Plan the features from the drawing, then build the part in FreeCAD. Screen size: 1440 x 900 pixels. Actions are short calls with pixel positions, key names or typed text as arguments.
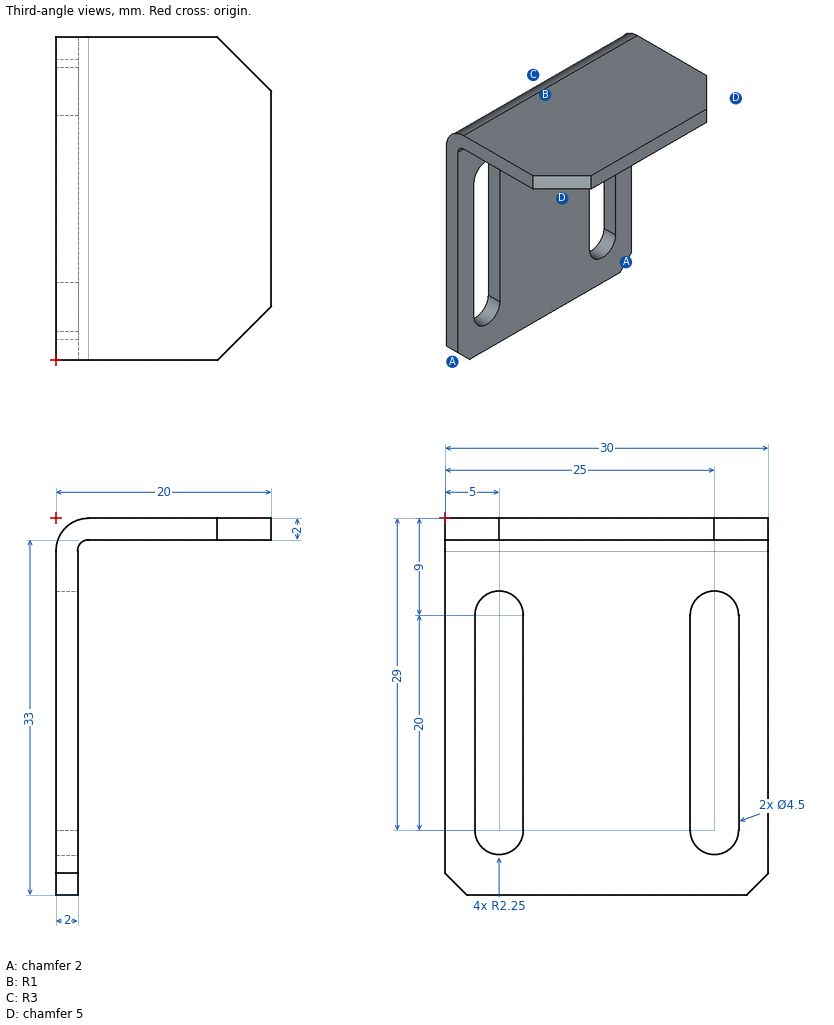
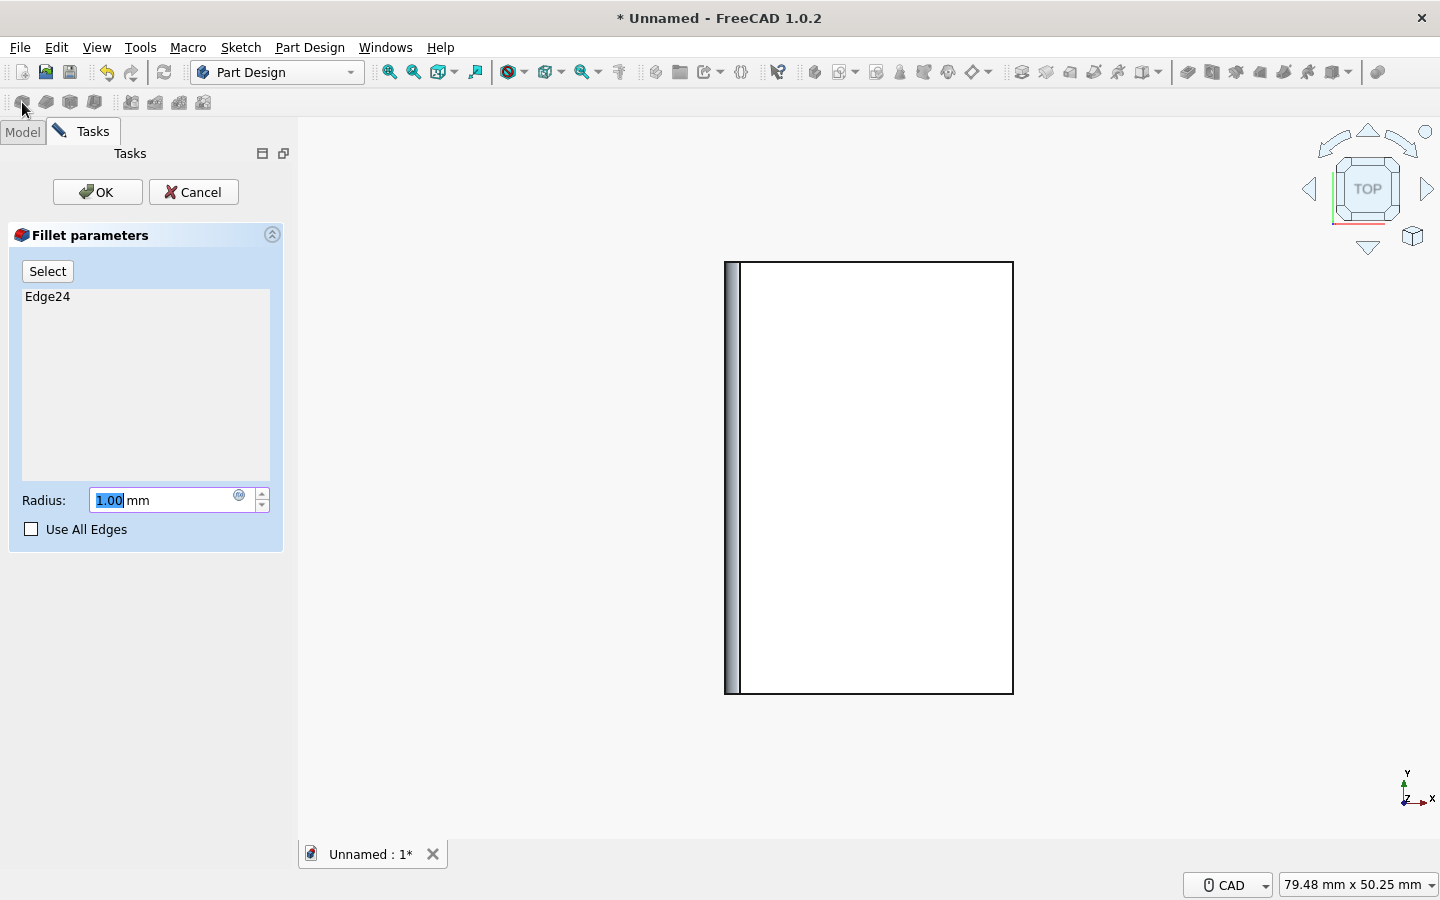
text(3)
key(Tab)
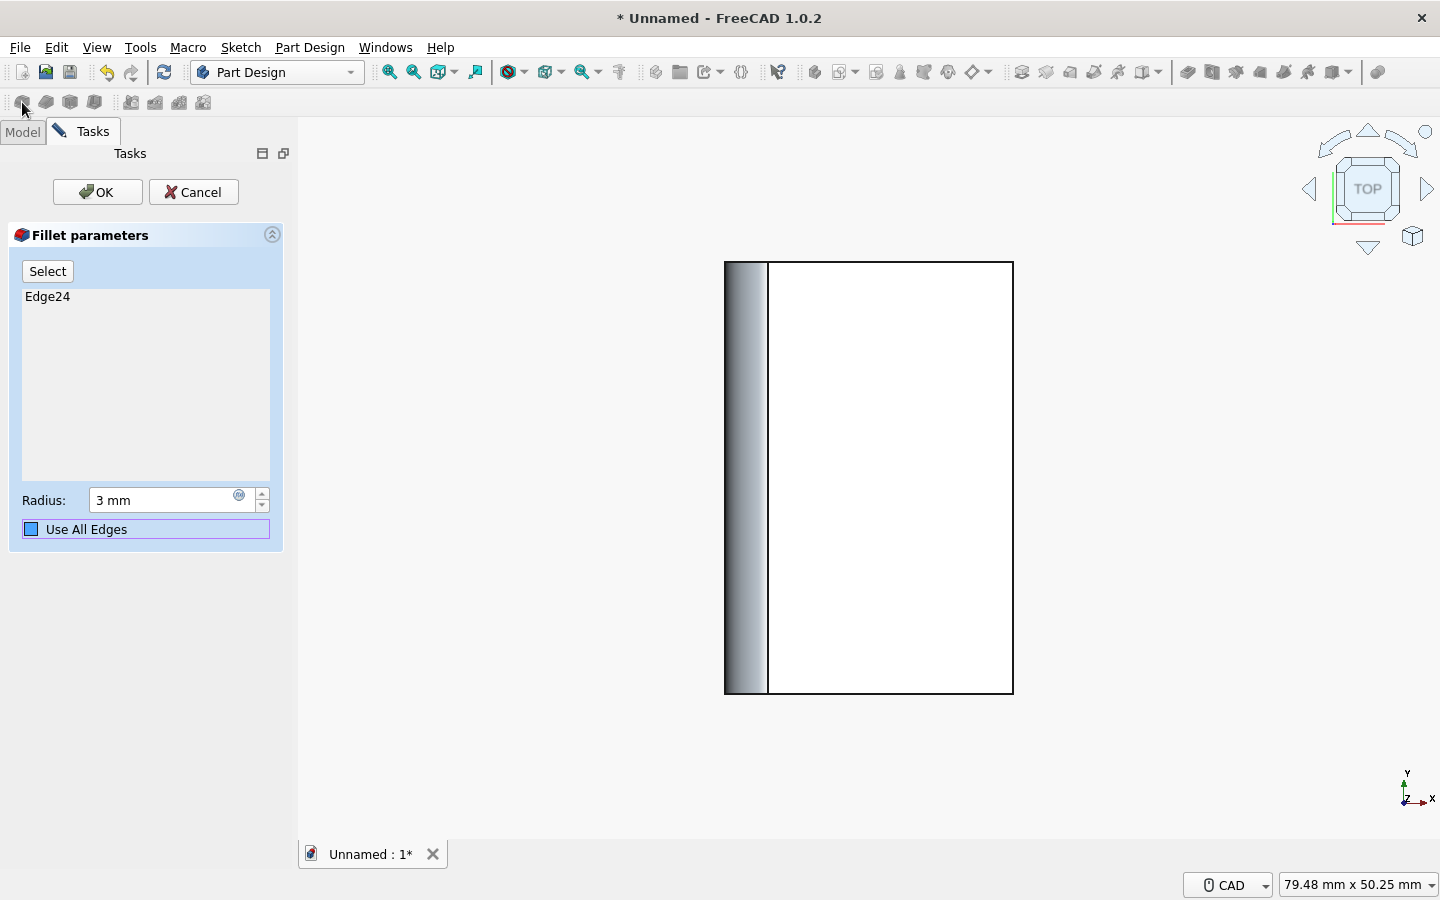
click(98, 192)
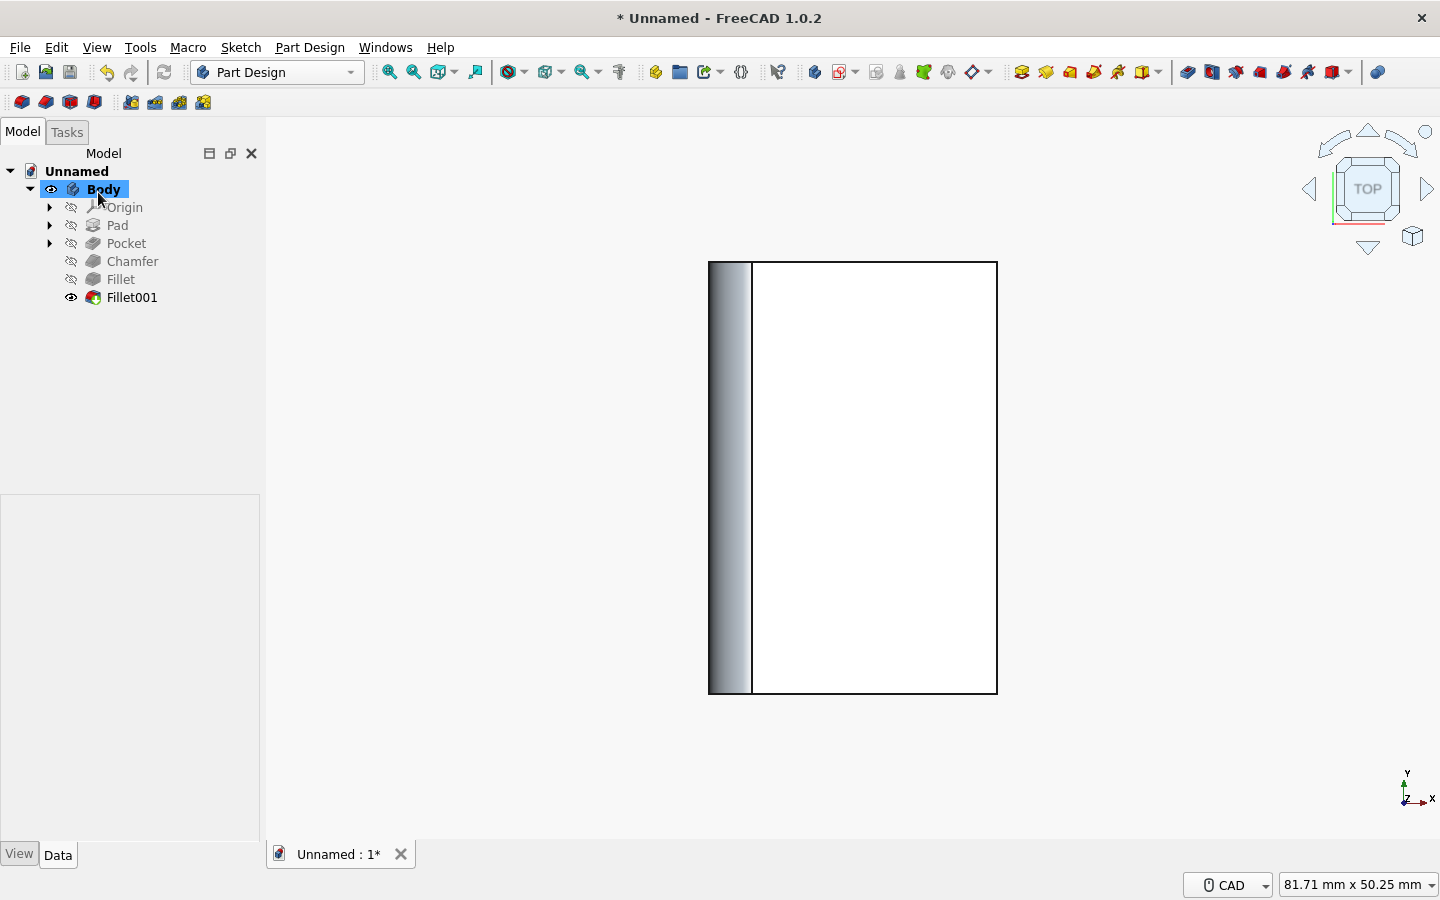
key(0)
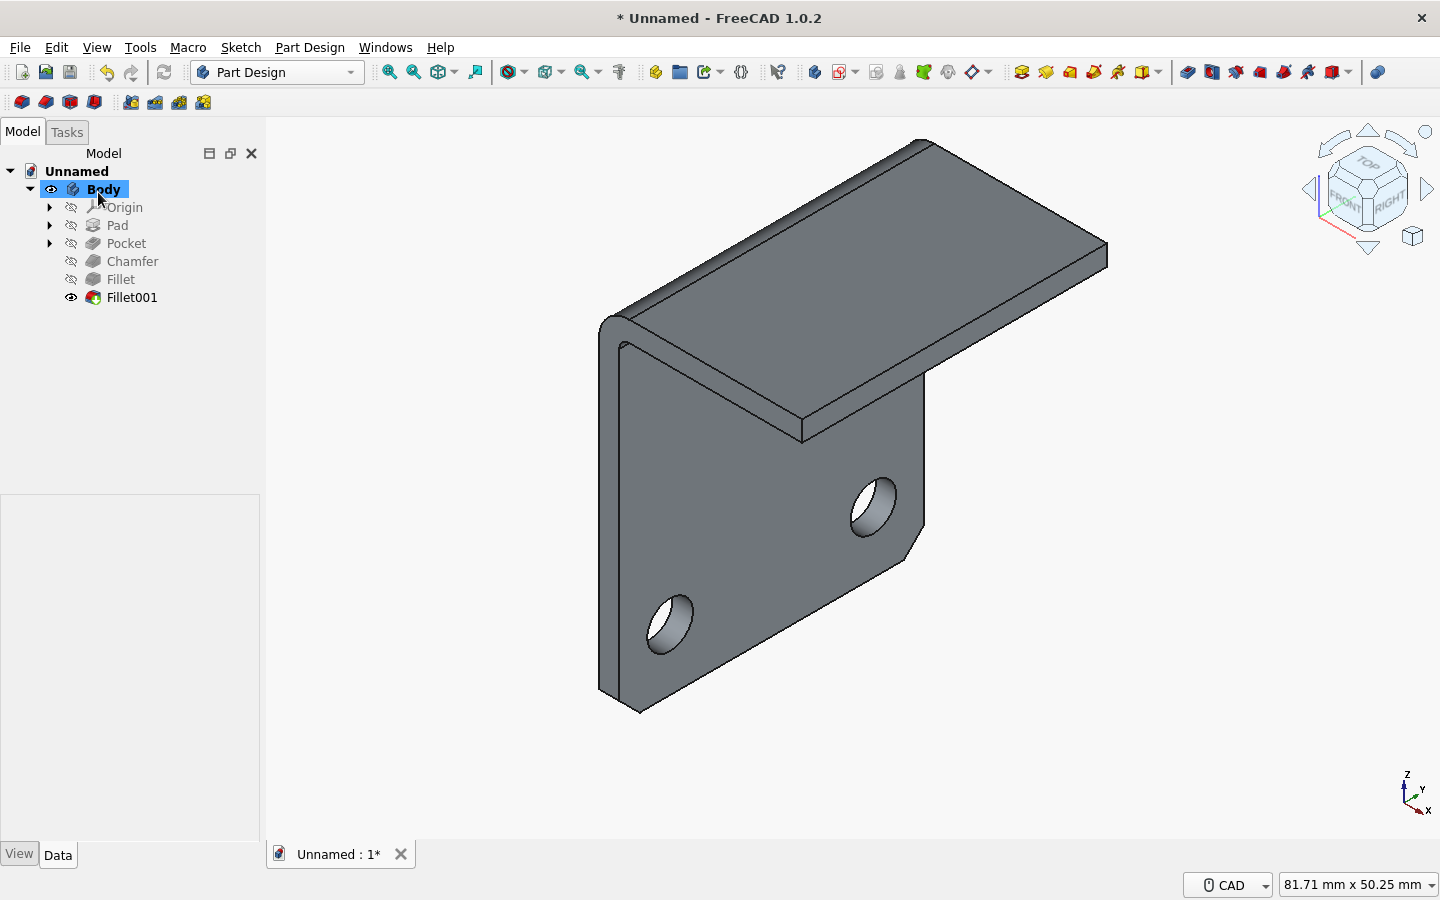
click(802, 430)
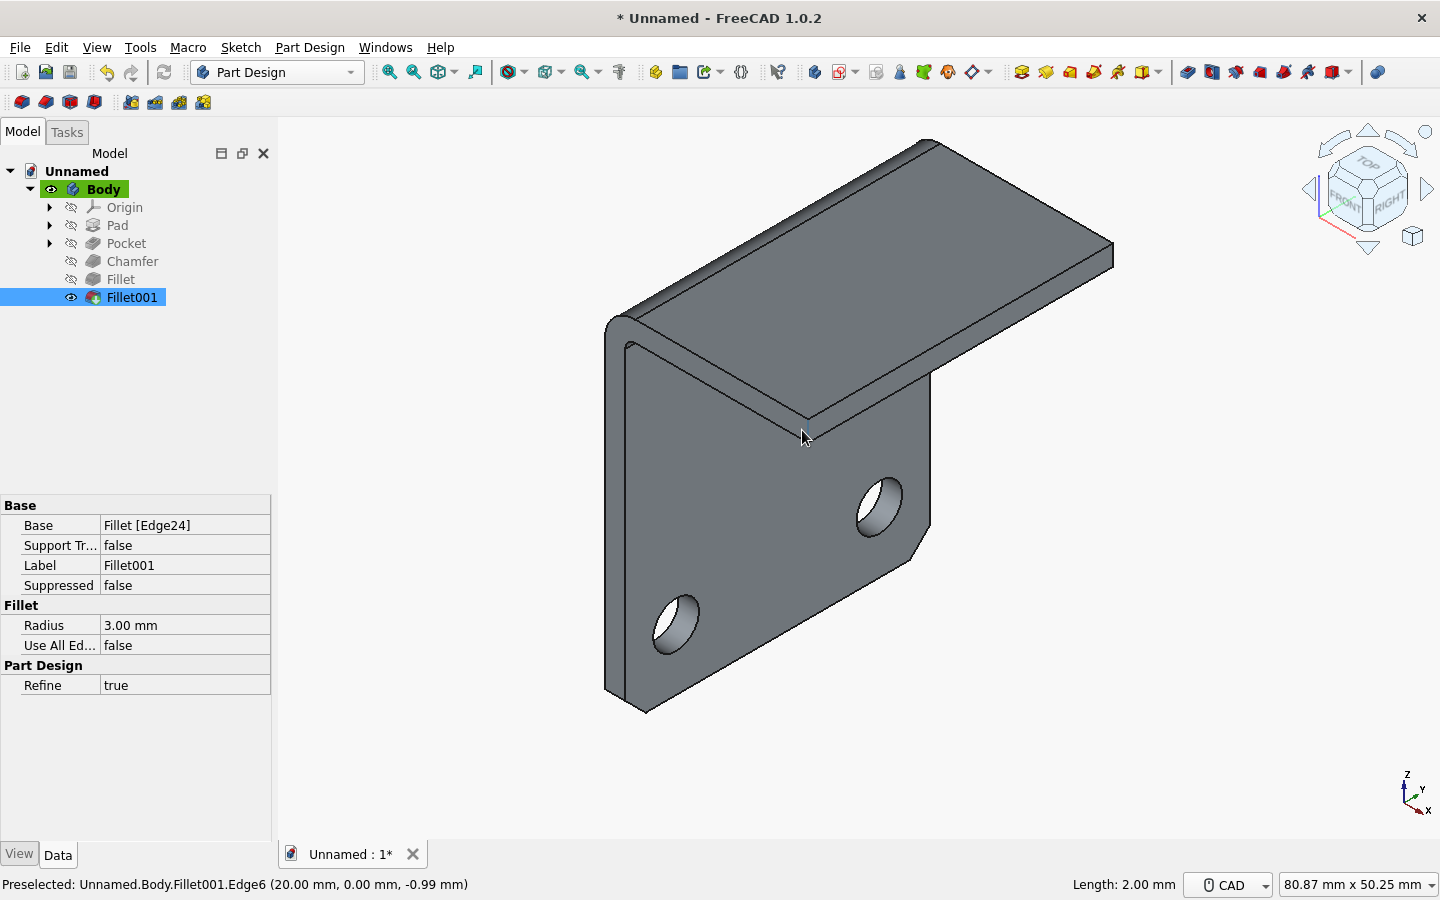
key(2)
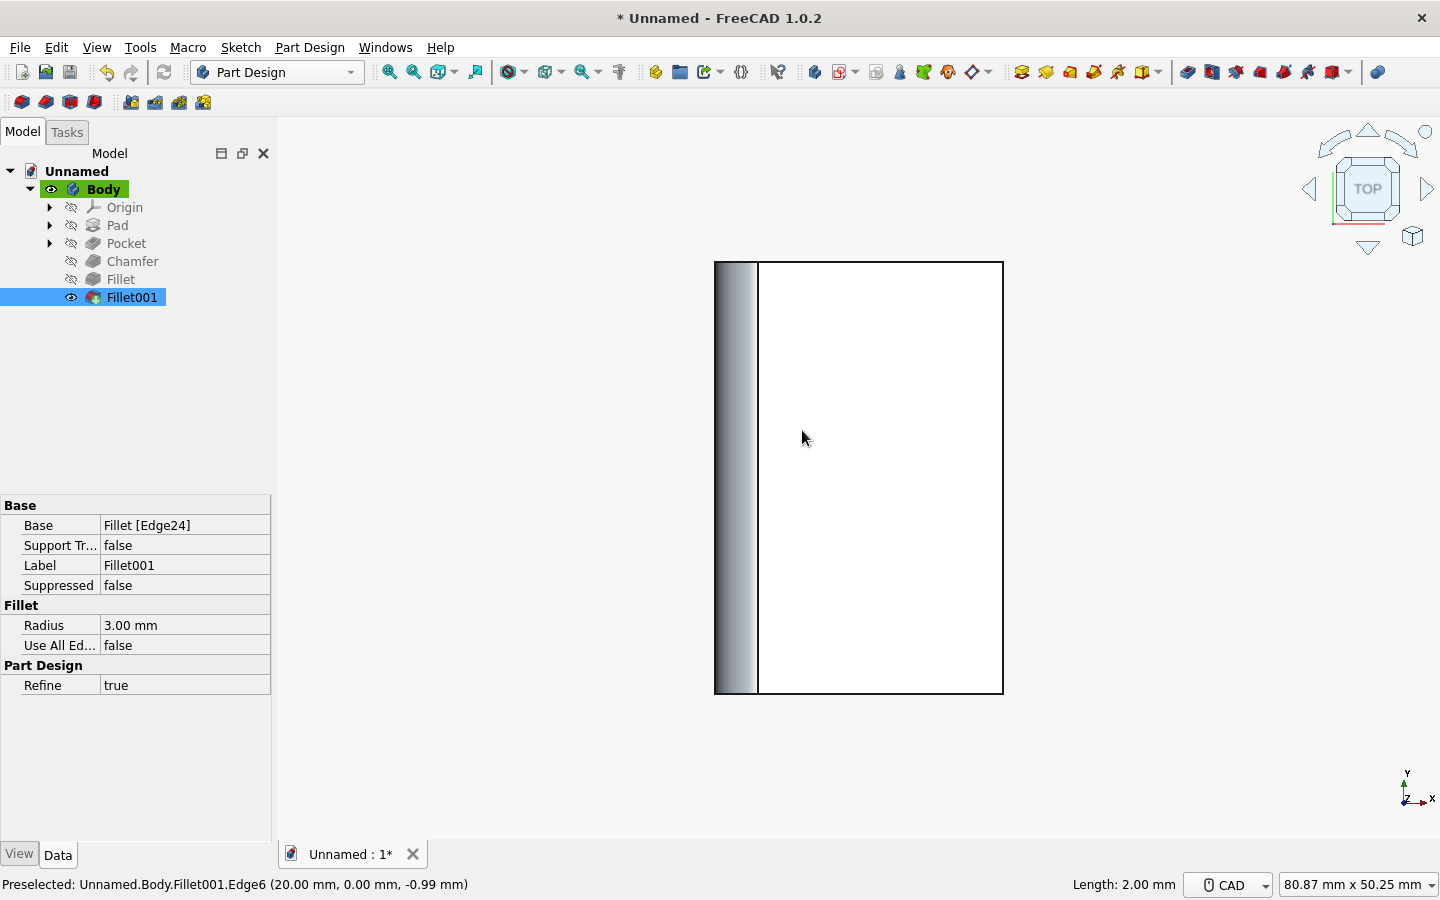
key(1)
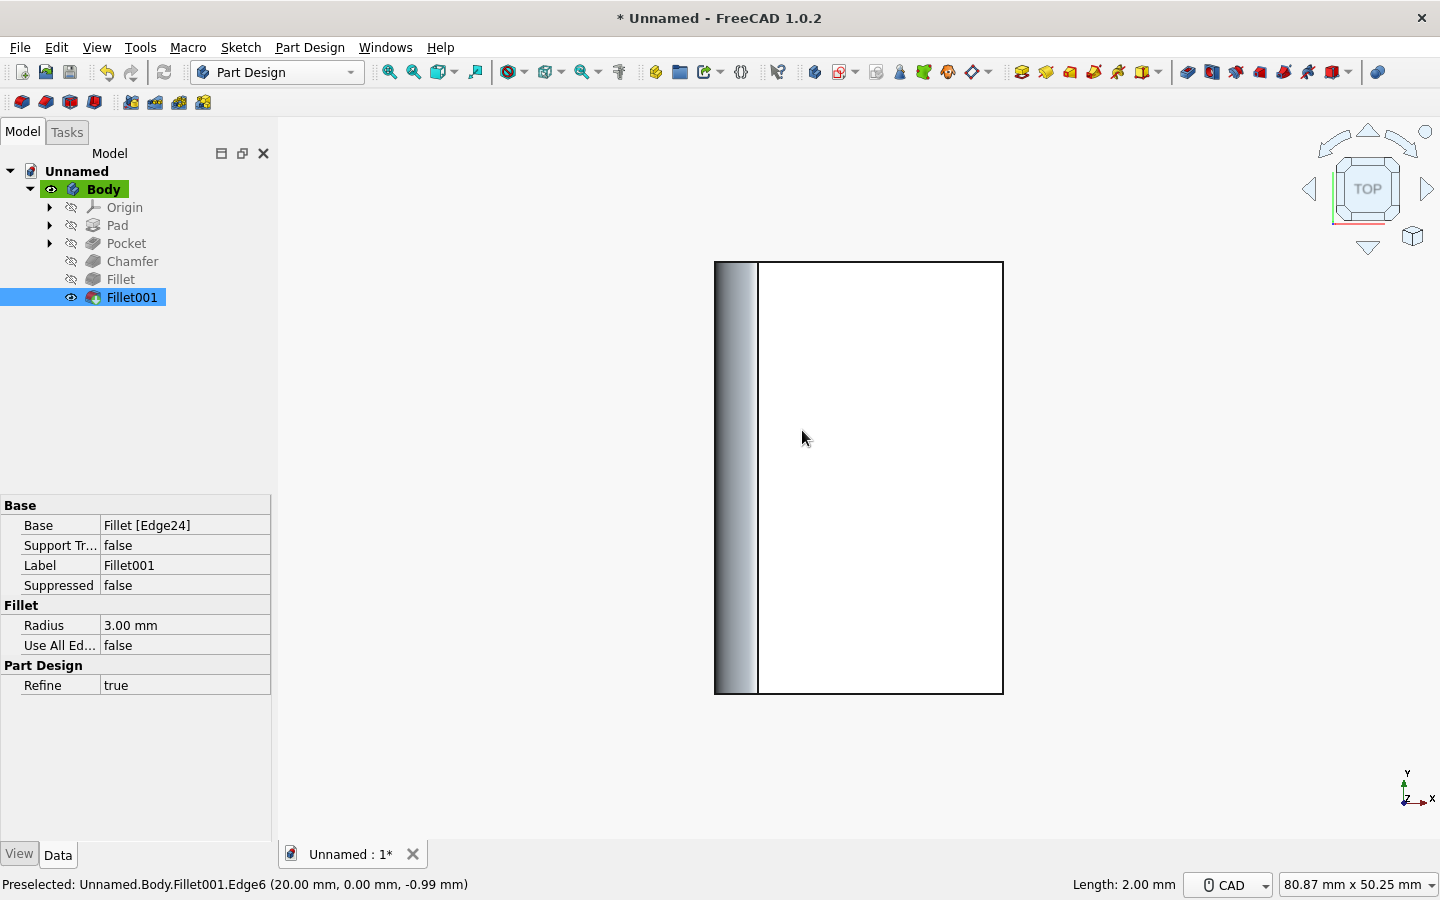
key(3)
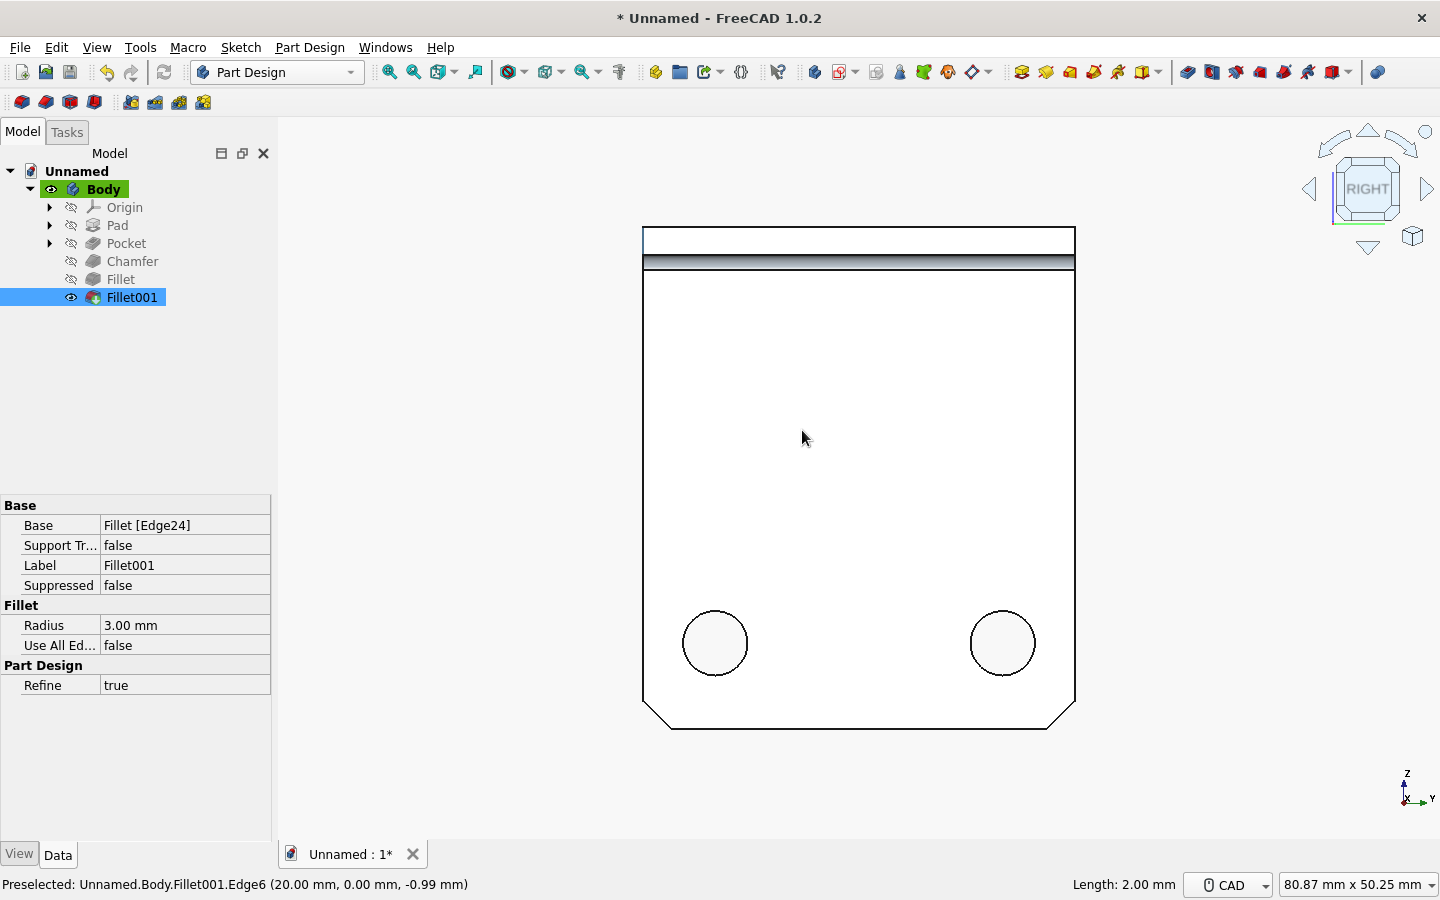
click(1075, 240, ctrl)